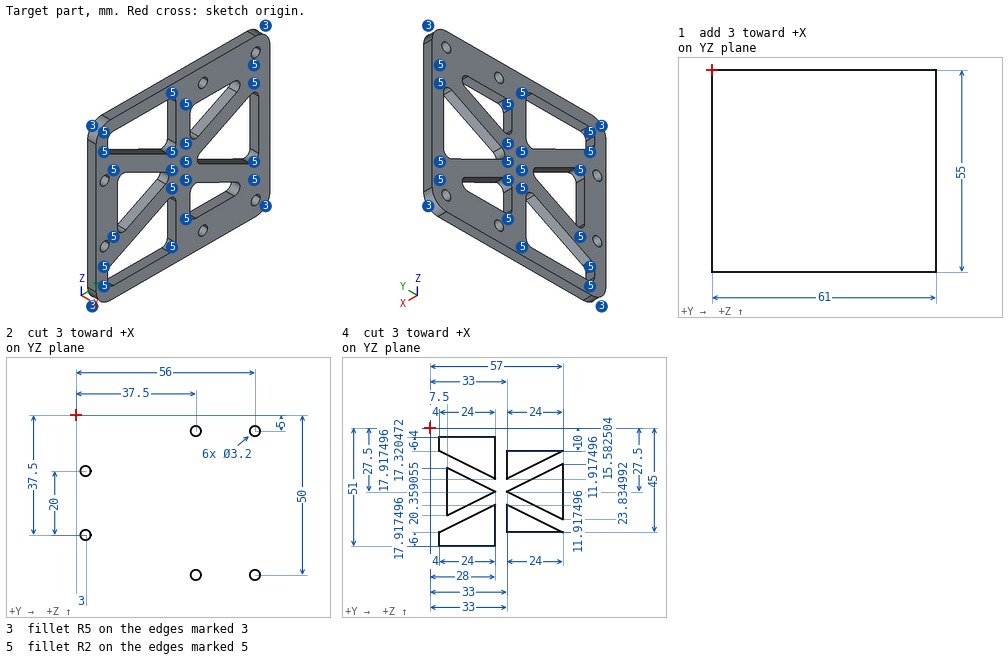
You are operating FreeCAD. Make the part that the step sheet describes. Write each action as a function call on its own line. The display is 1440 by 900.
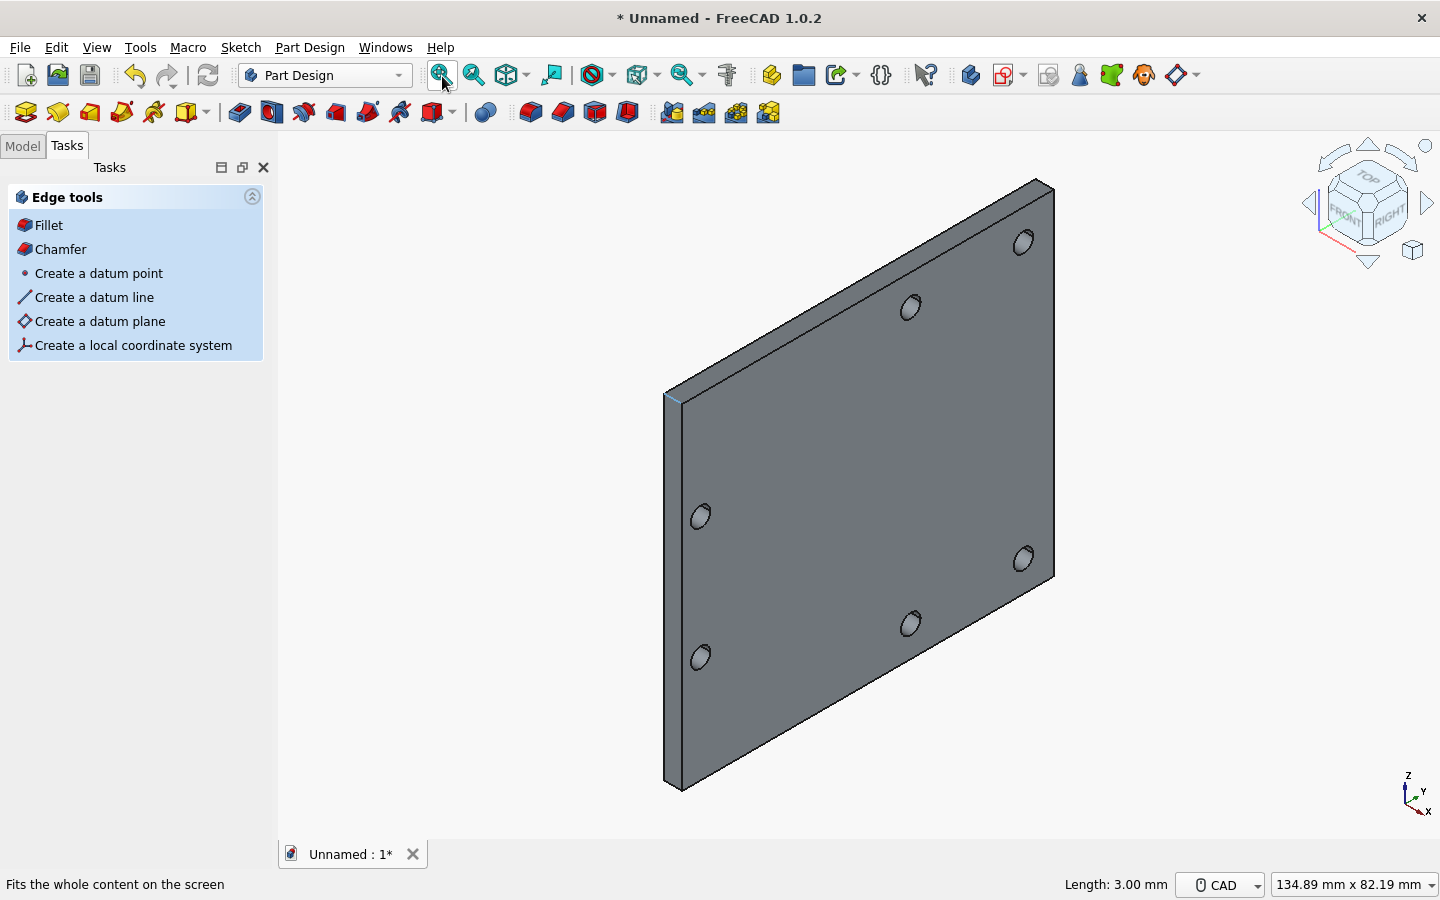
key(2)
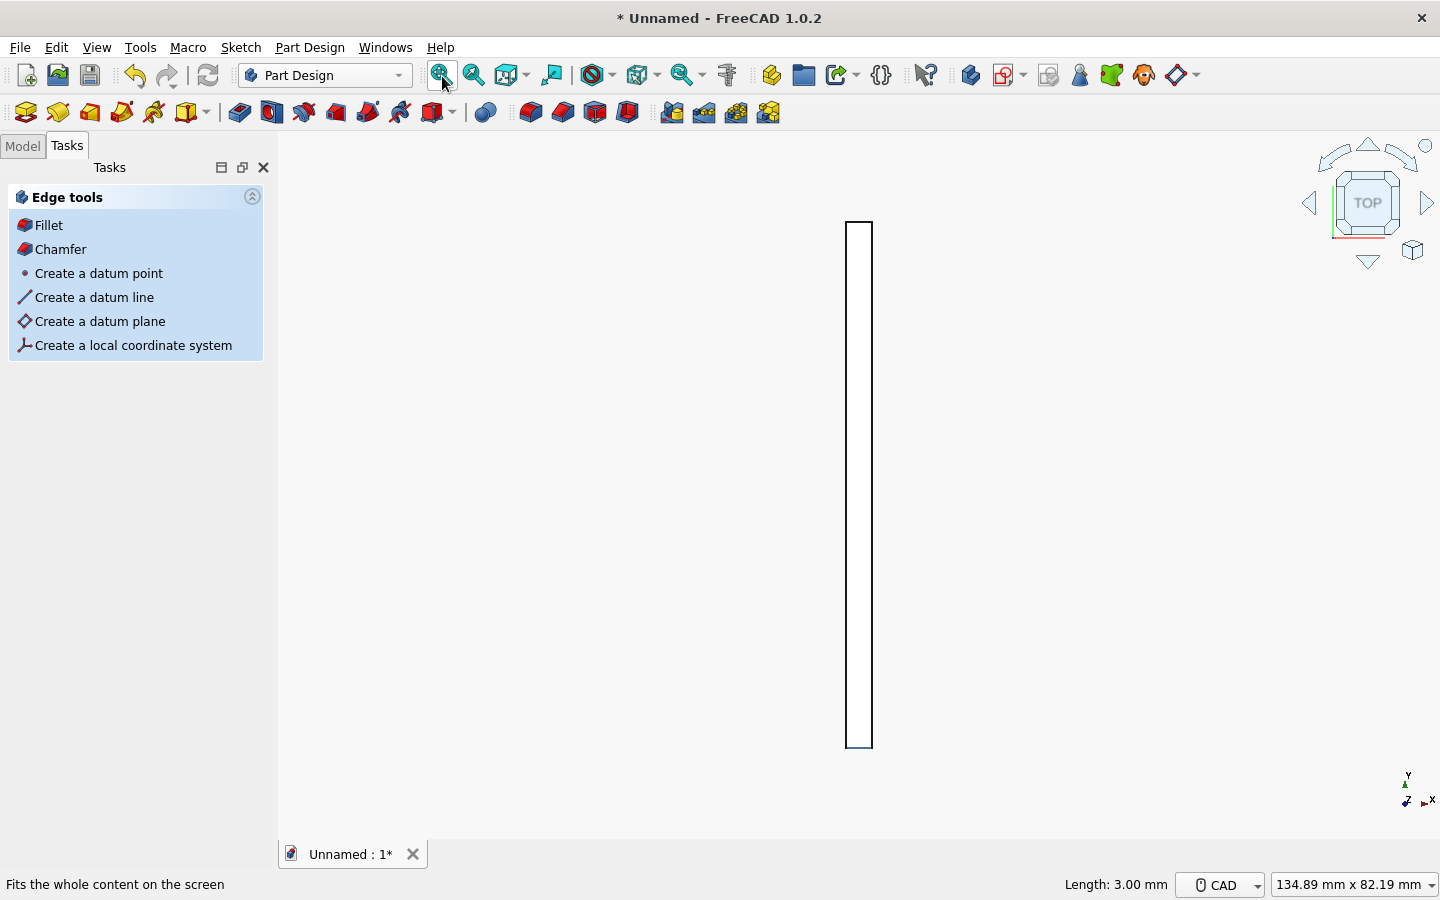
key(1)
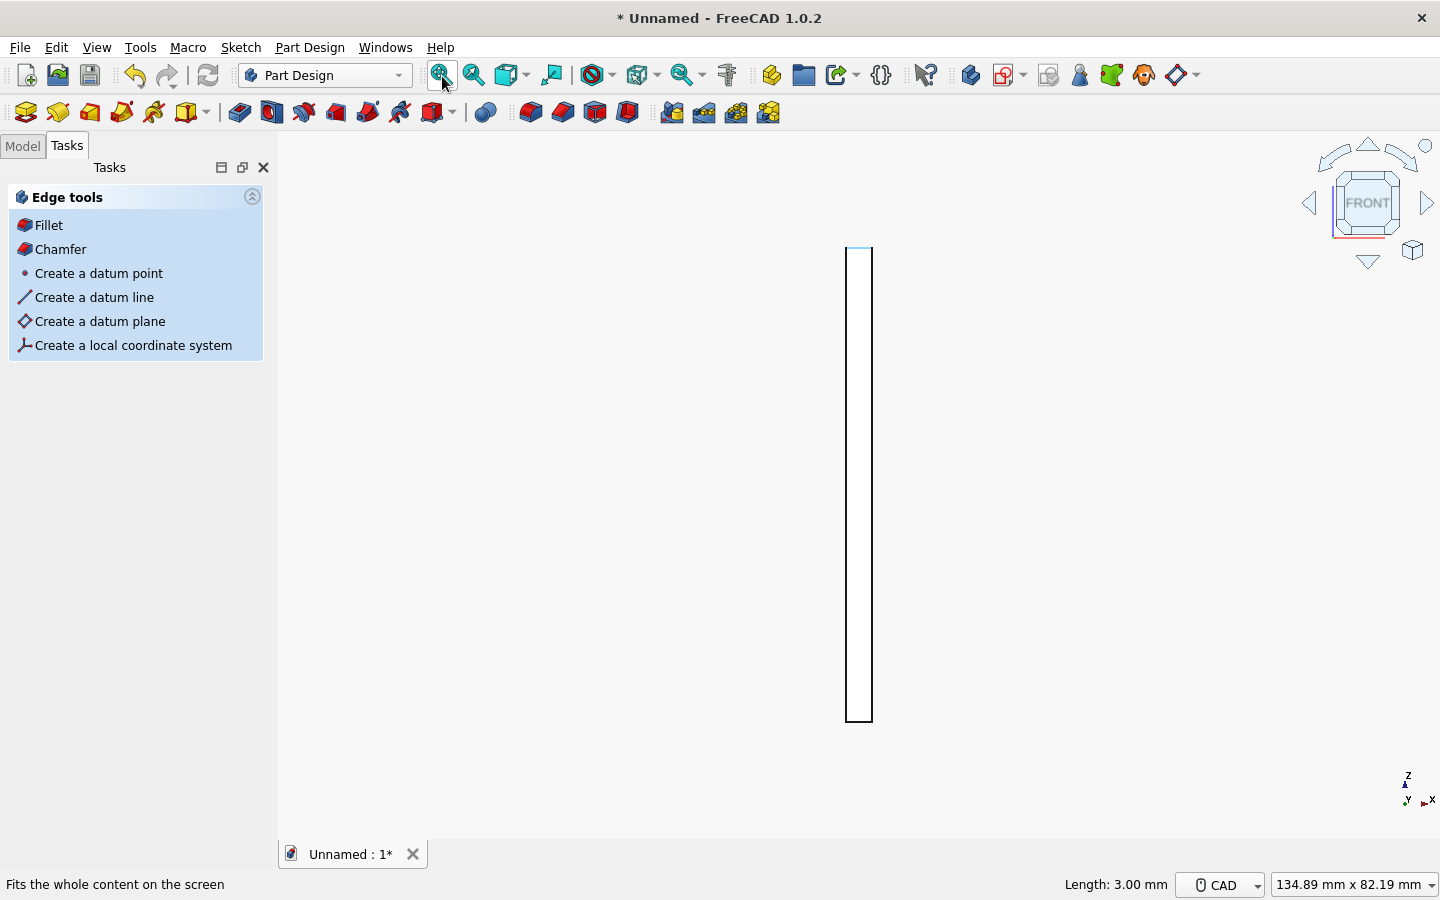
click(859, 721, ctrl)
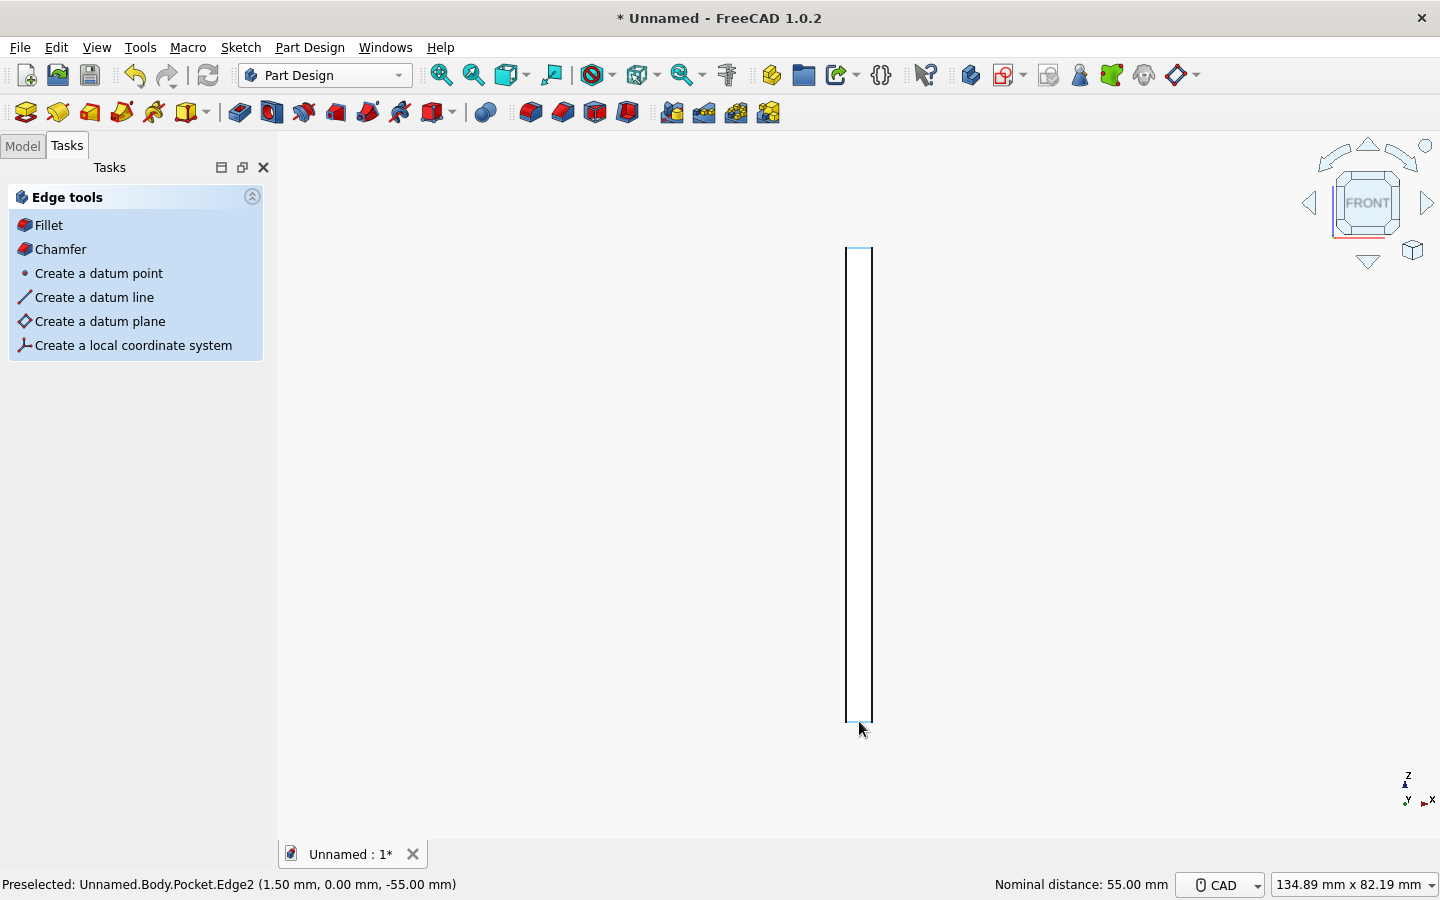
key(3)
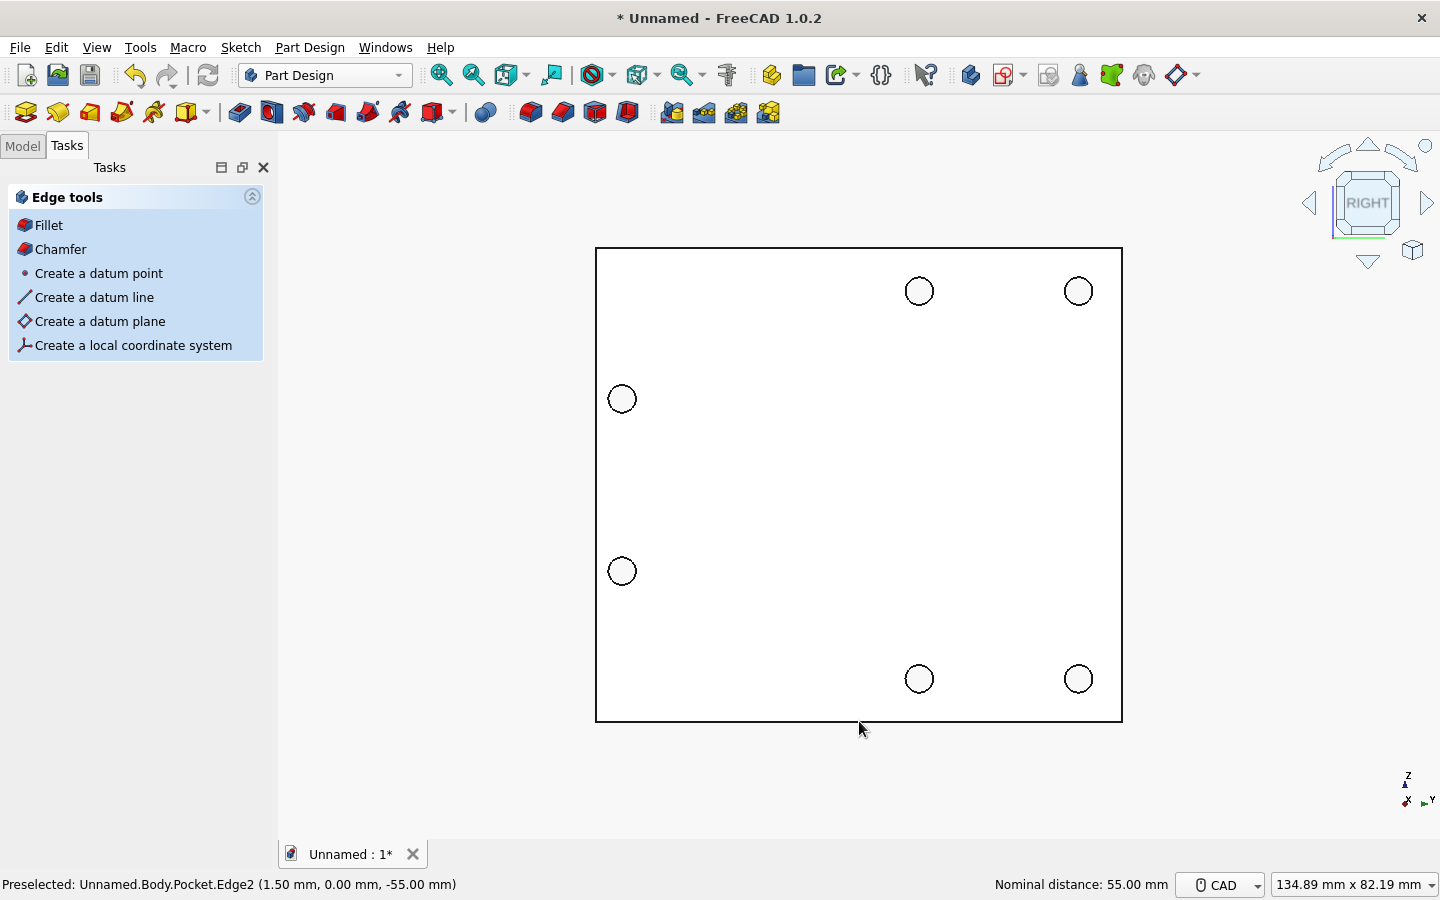
key(5)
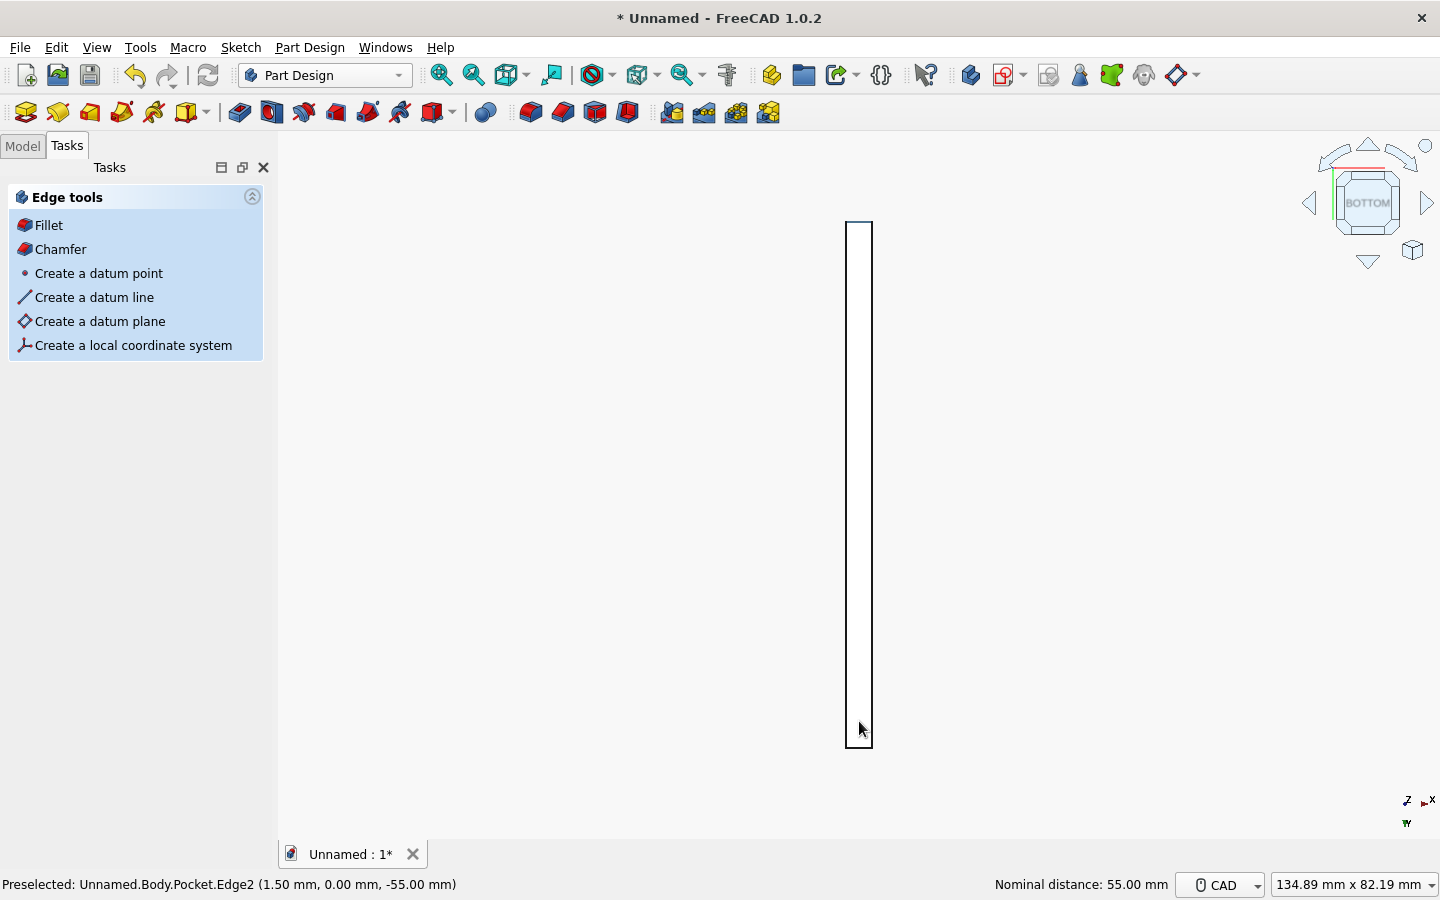
click(859, 747, ctrl)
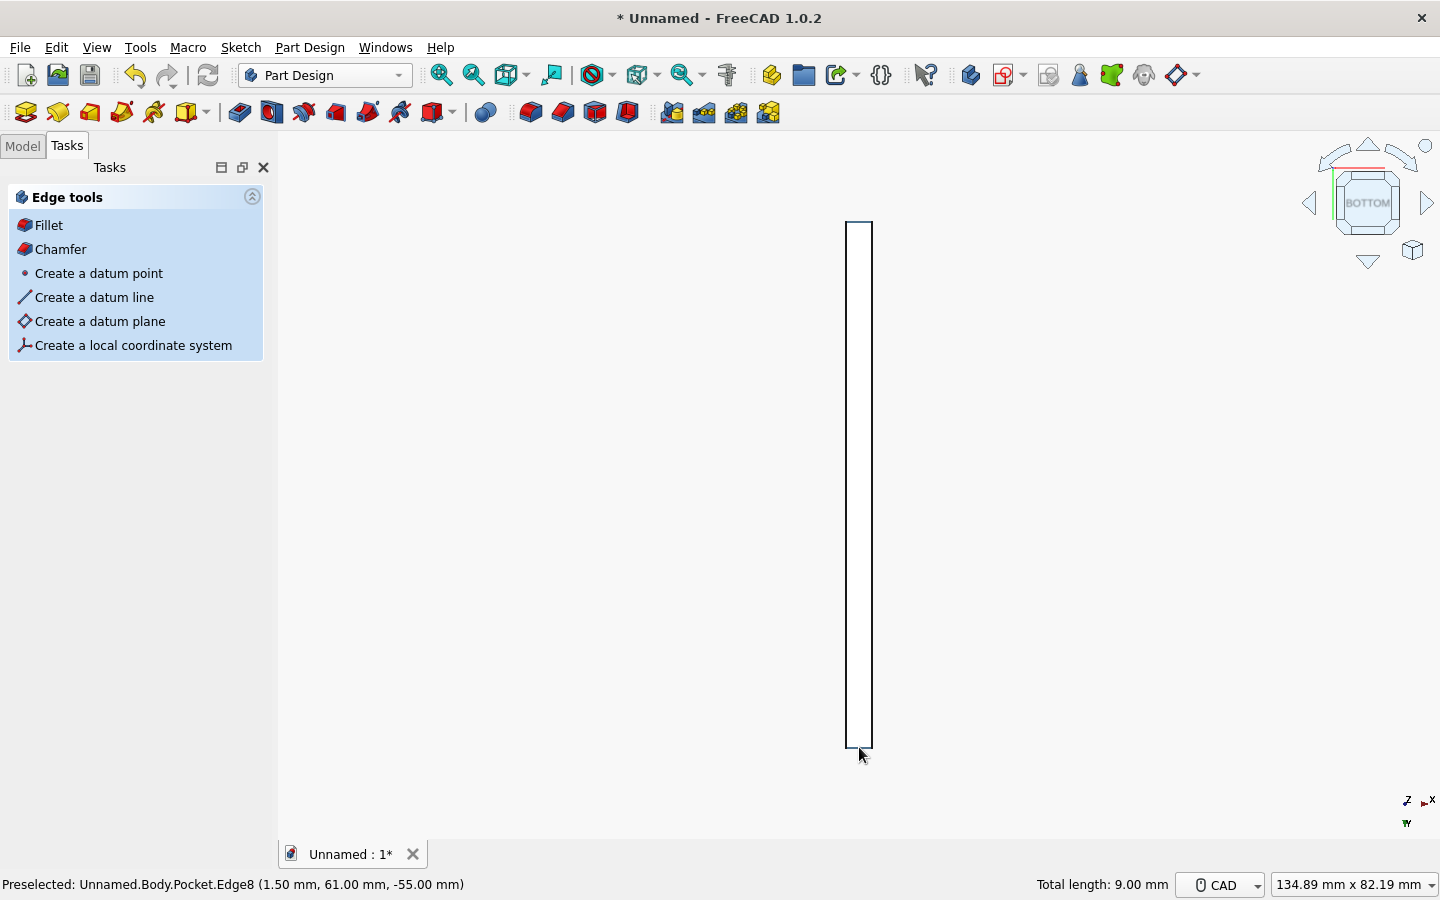
key(4)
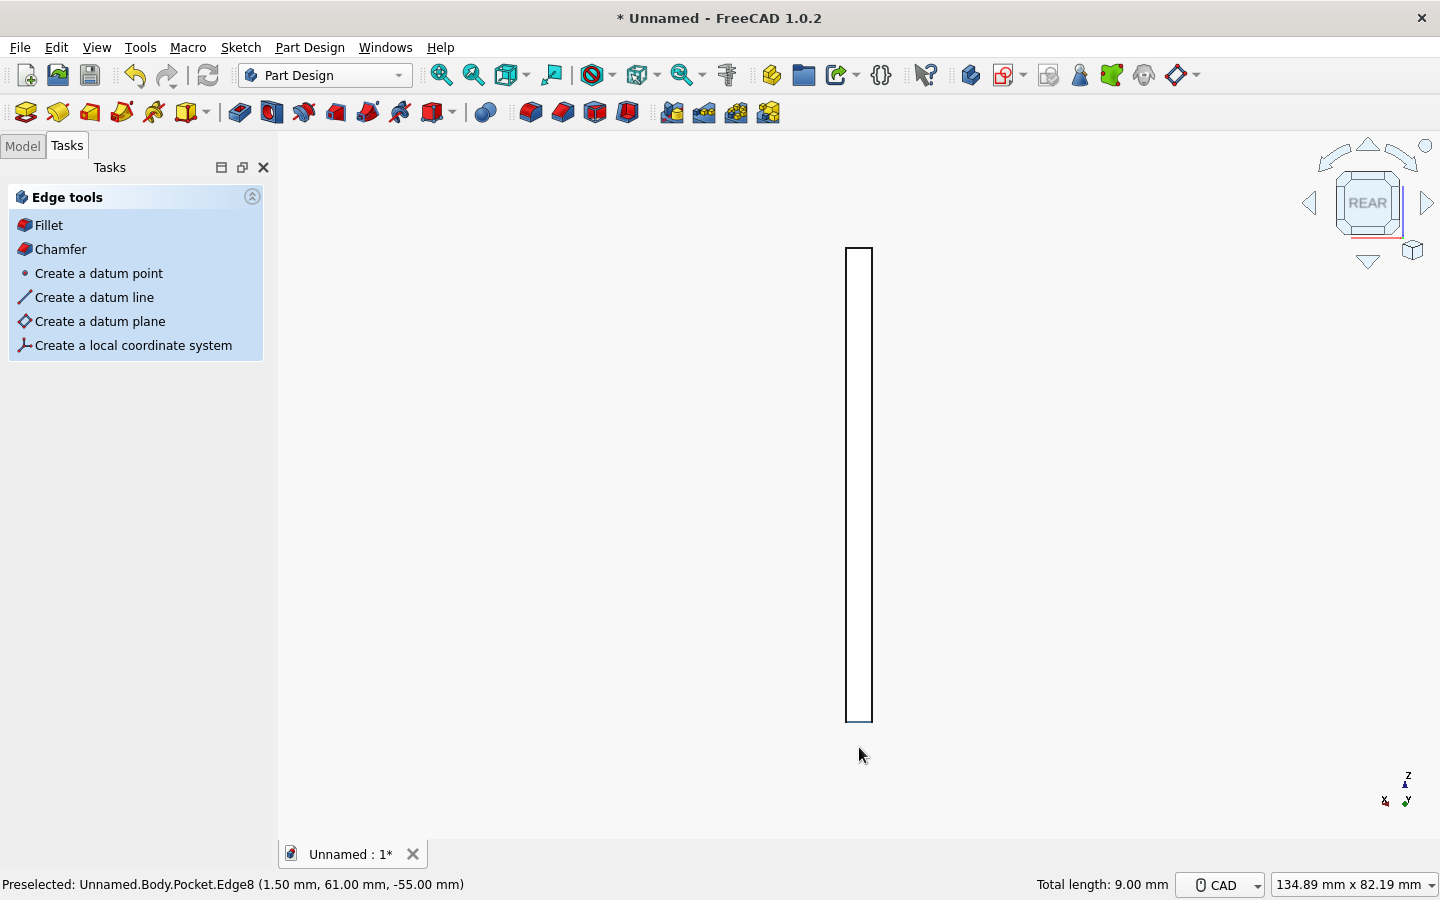
click(859, 247, ctrl)